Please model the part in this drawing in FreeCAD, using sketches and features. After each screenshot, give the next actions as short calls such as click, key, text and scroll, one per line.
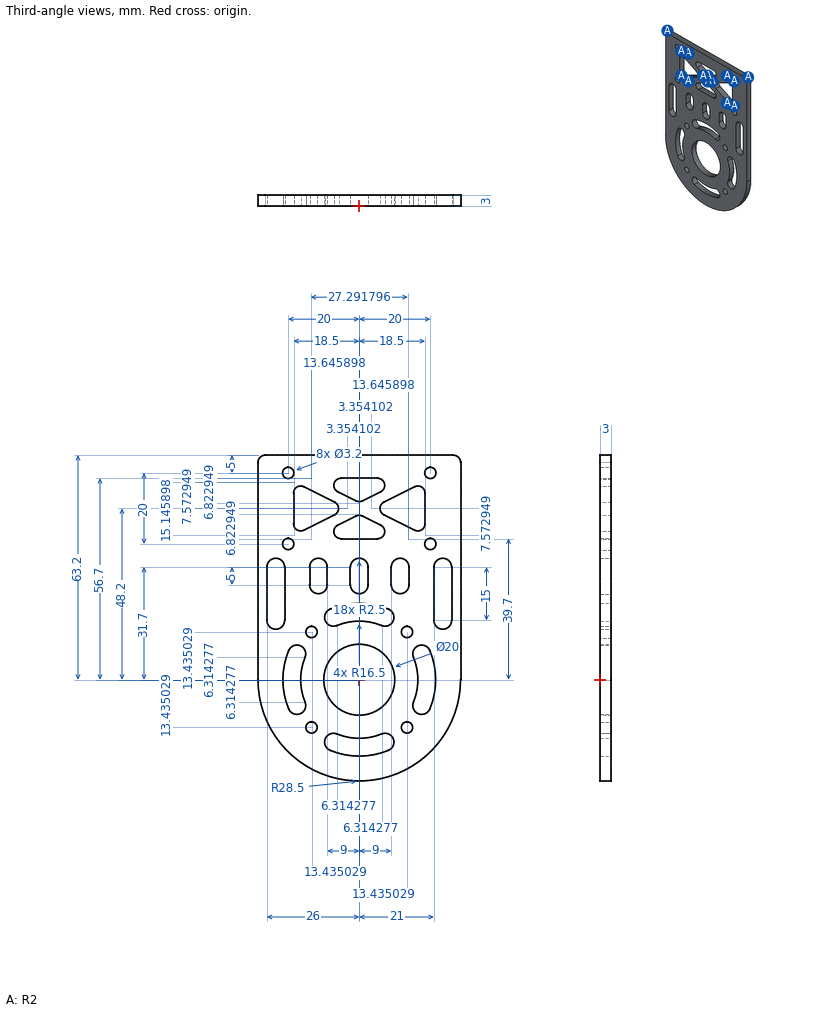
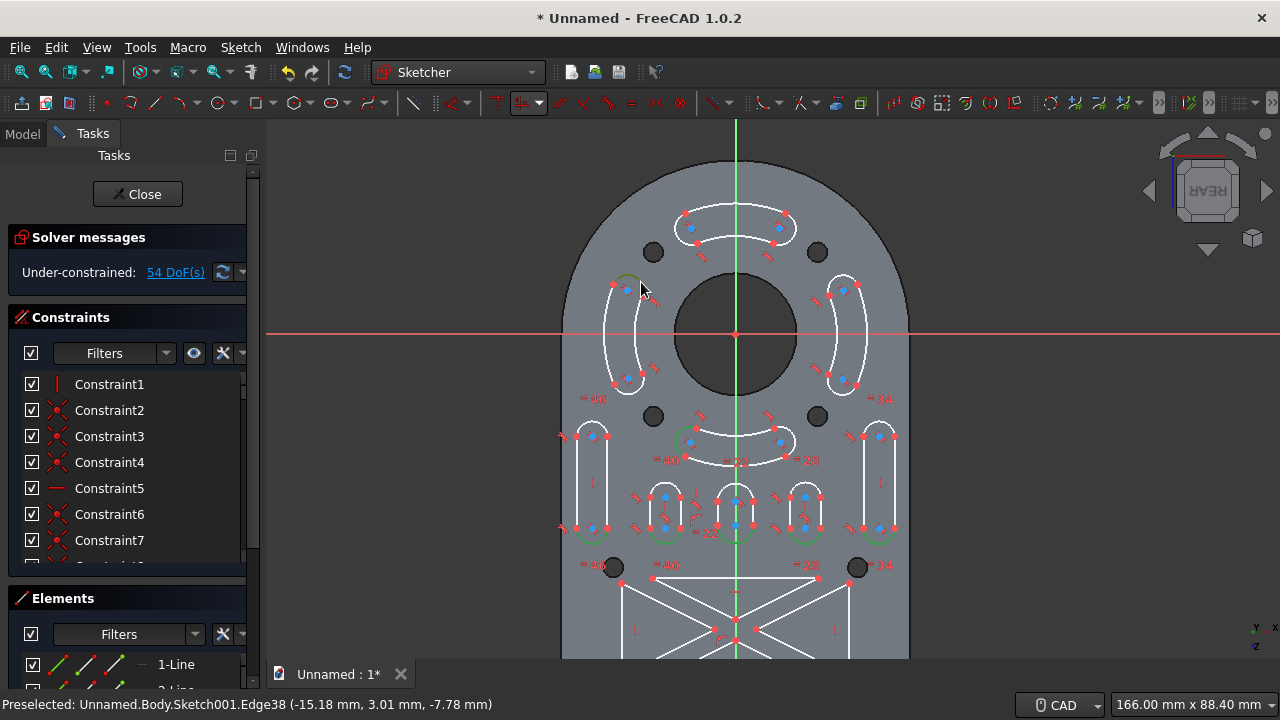
click(830, 388)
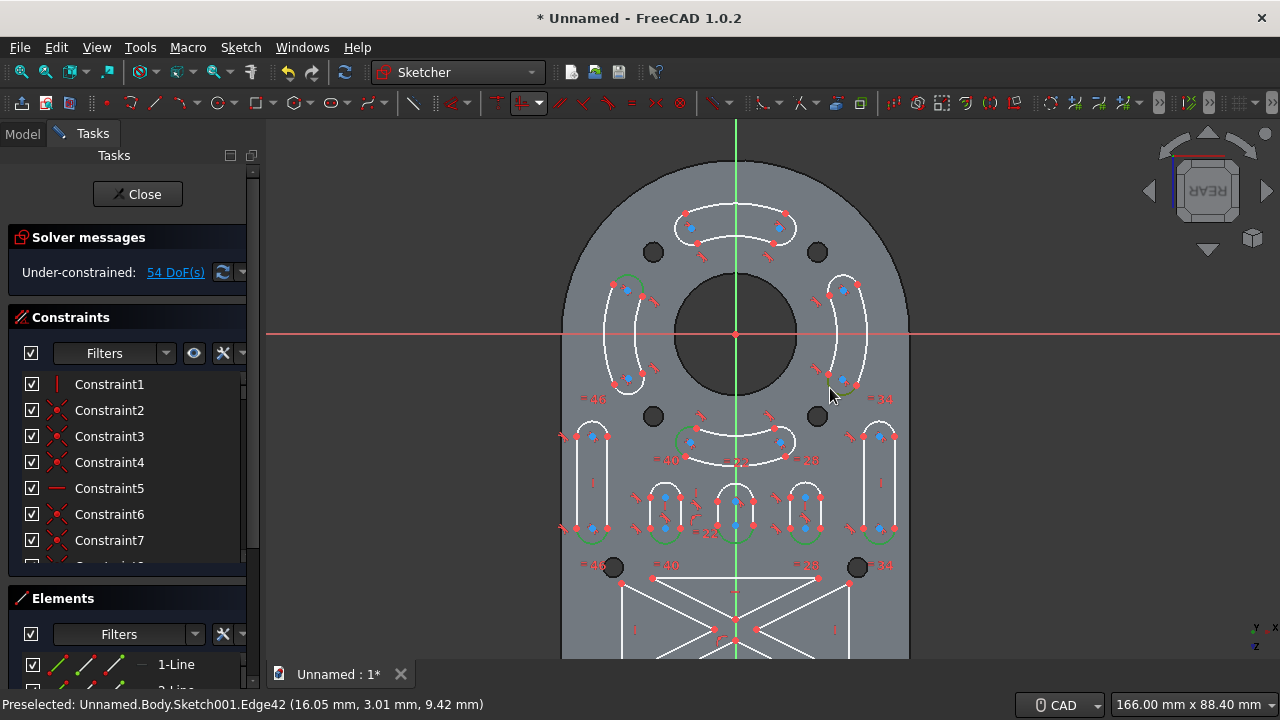
click(788, 242)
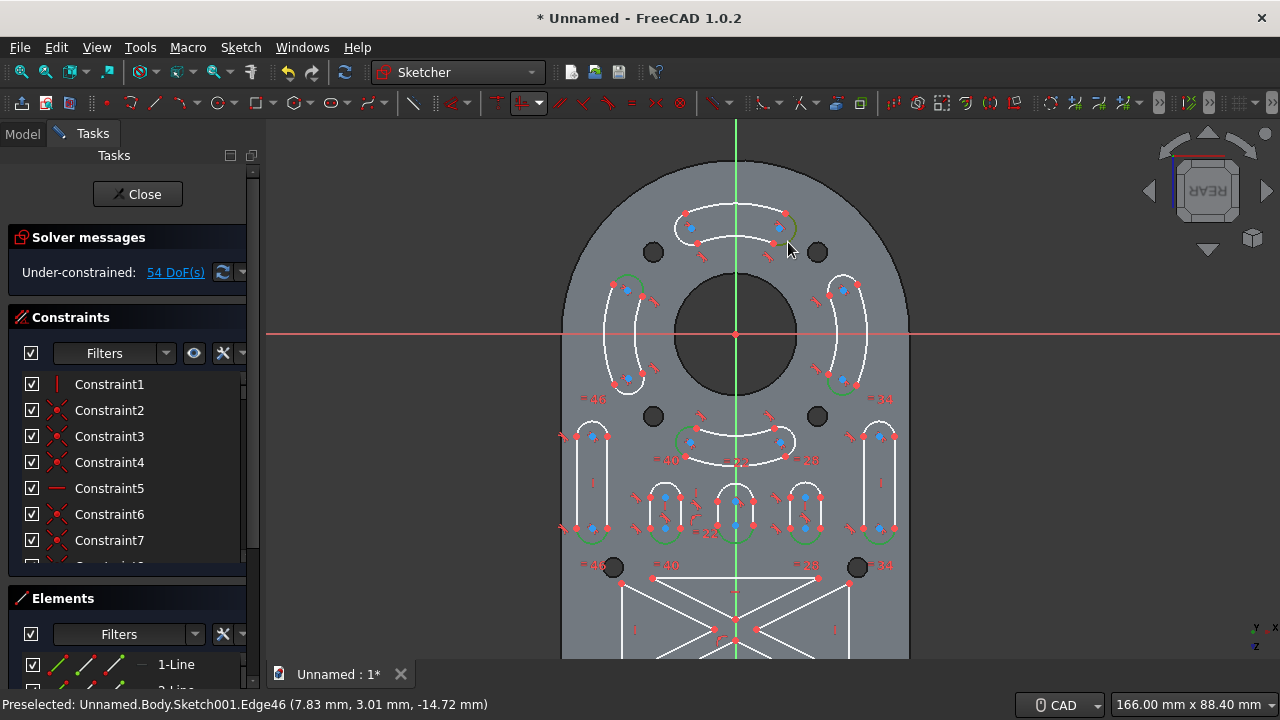
key(e)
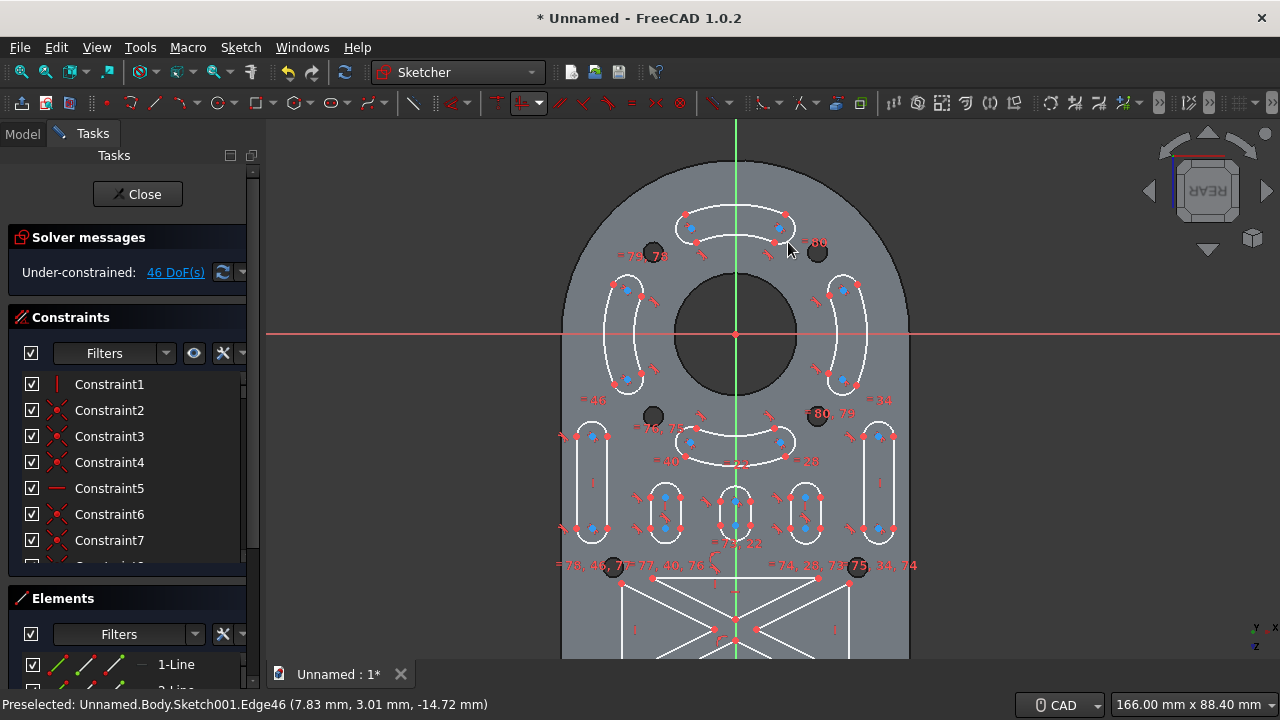
click(720, 435)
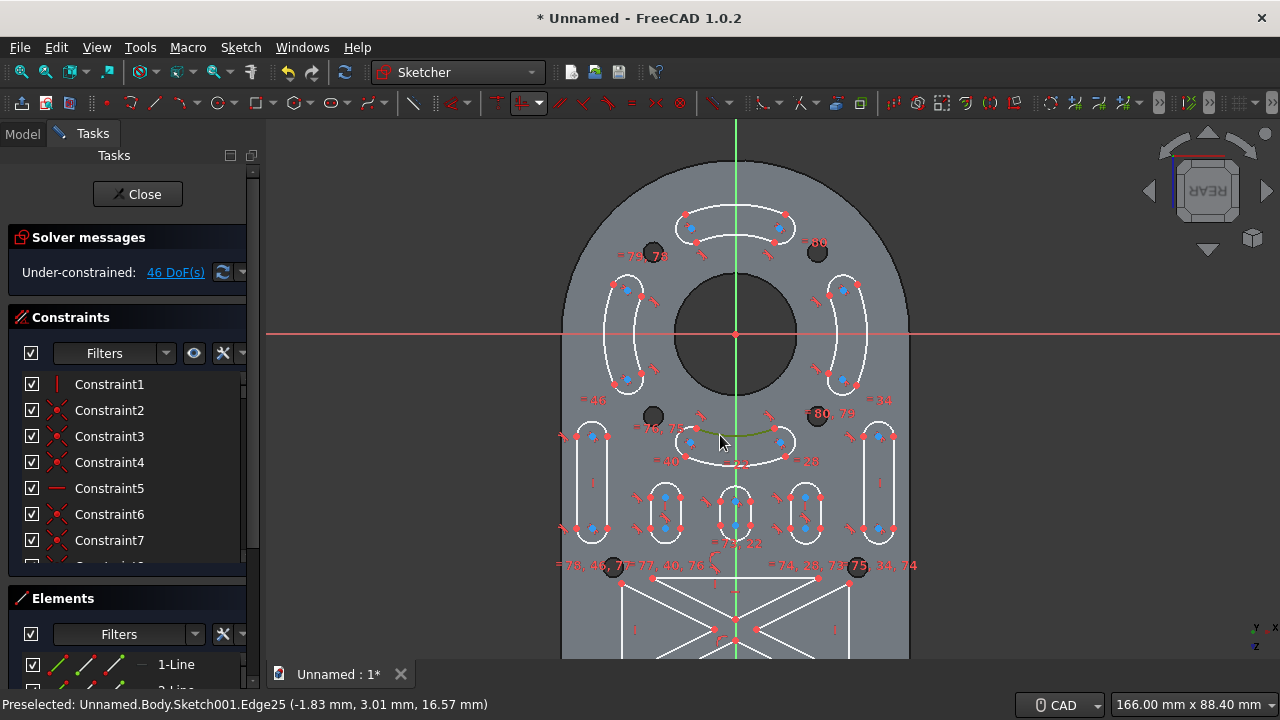
click(635, 319)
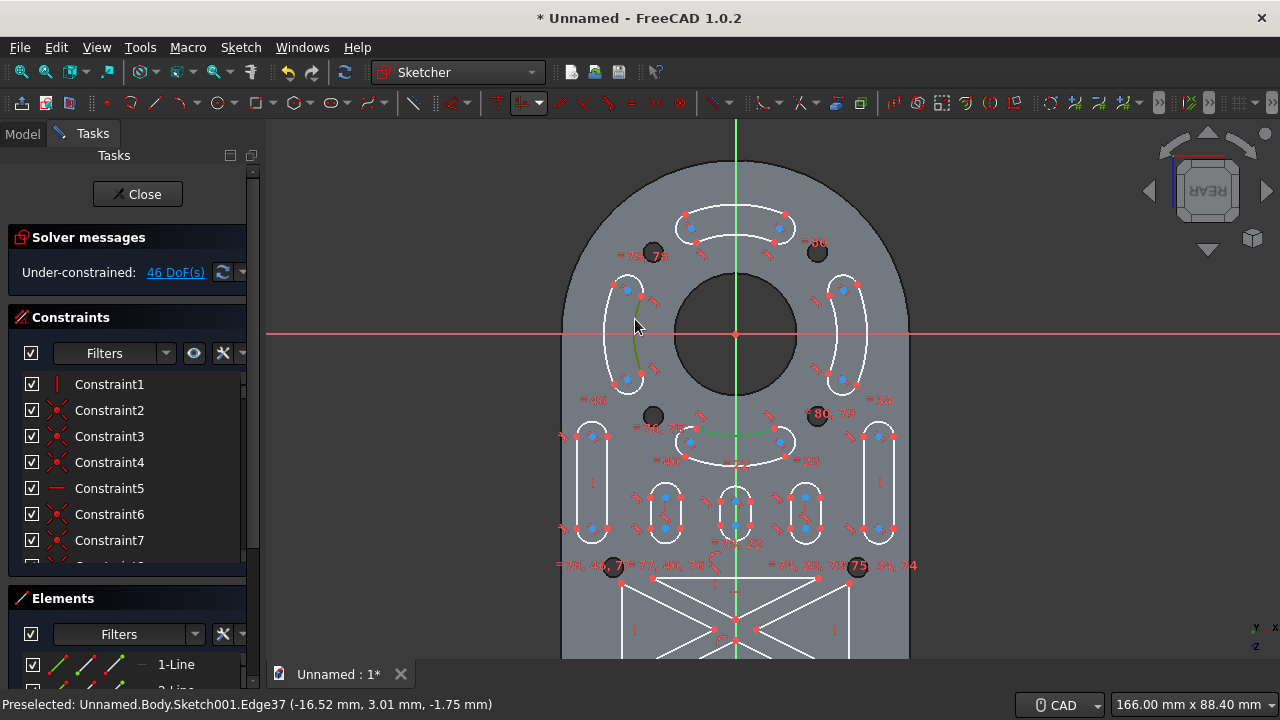
click(836, 351)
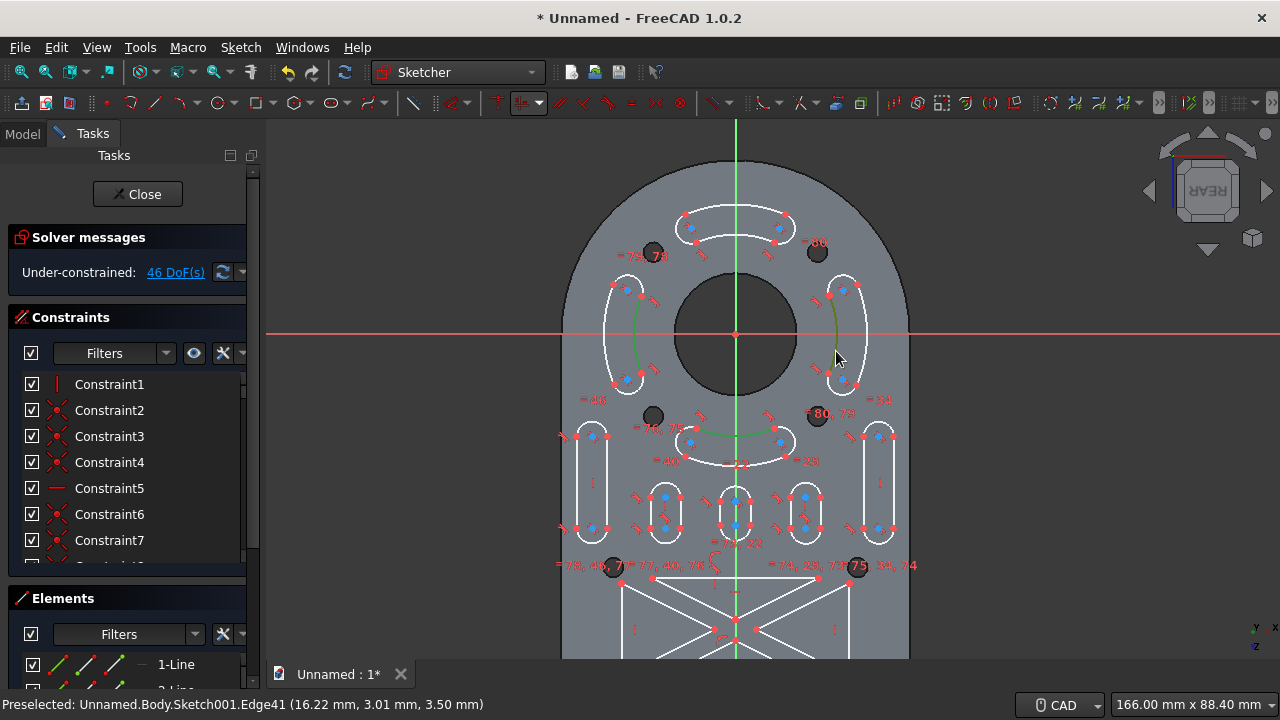
click(751, 236)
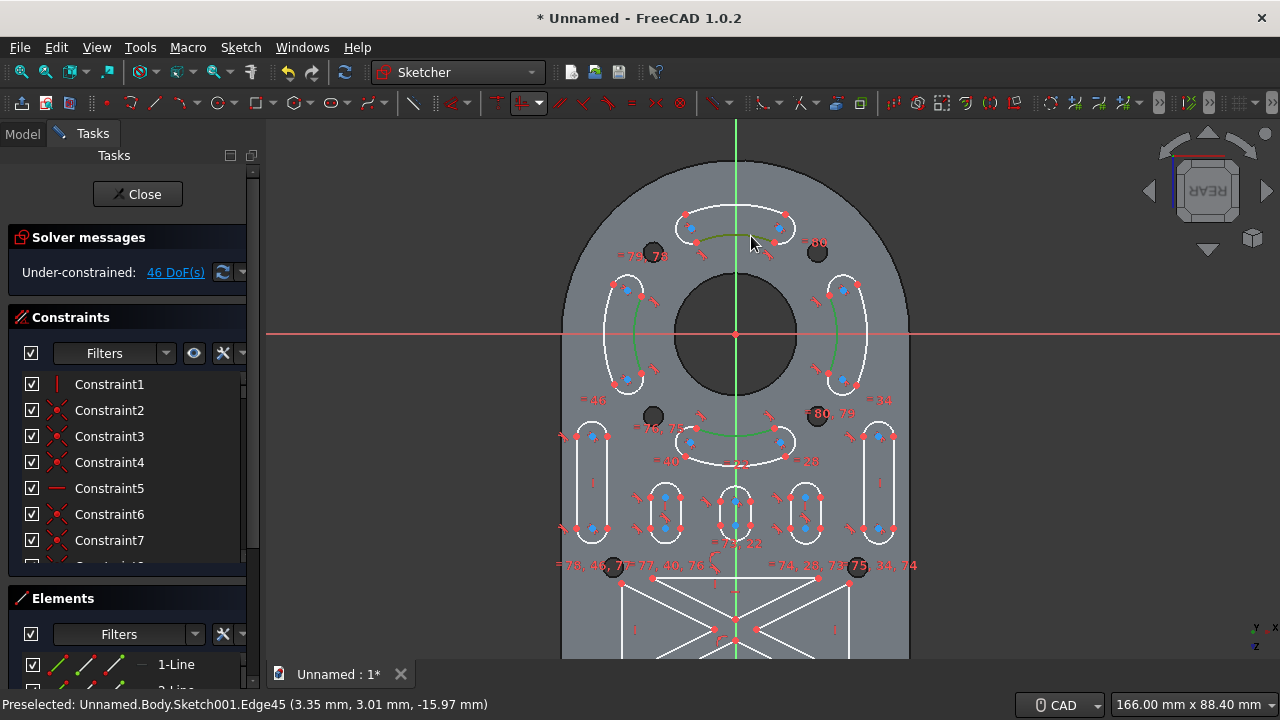
click(632, 104)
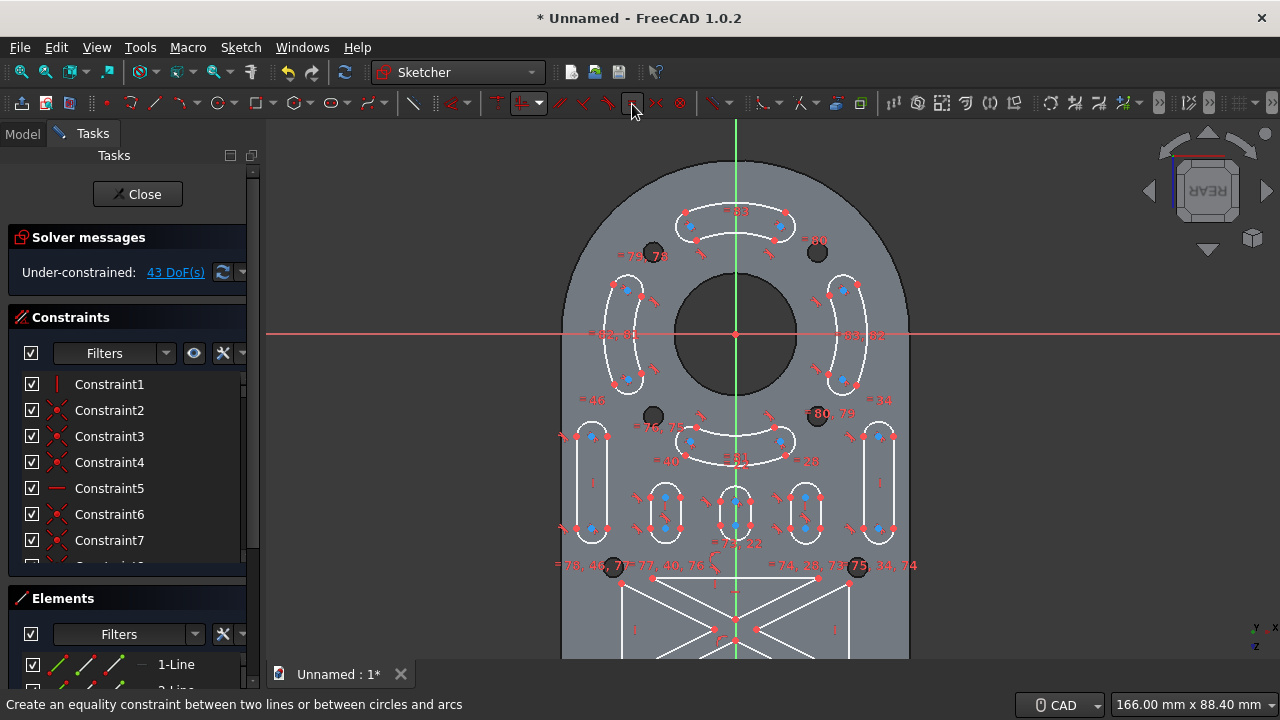
click(452, 104)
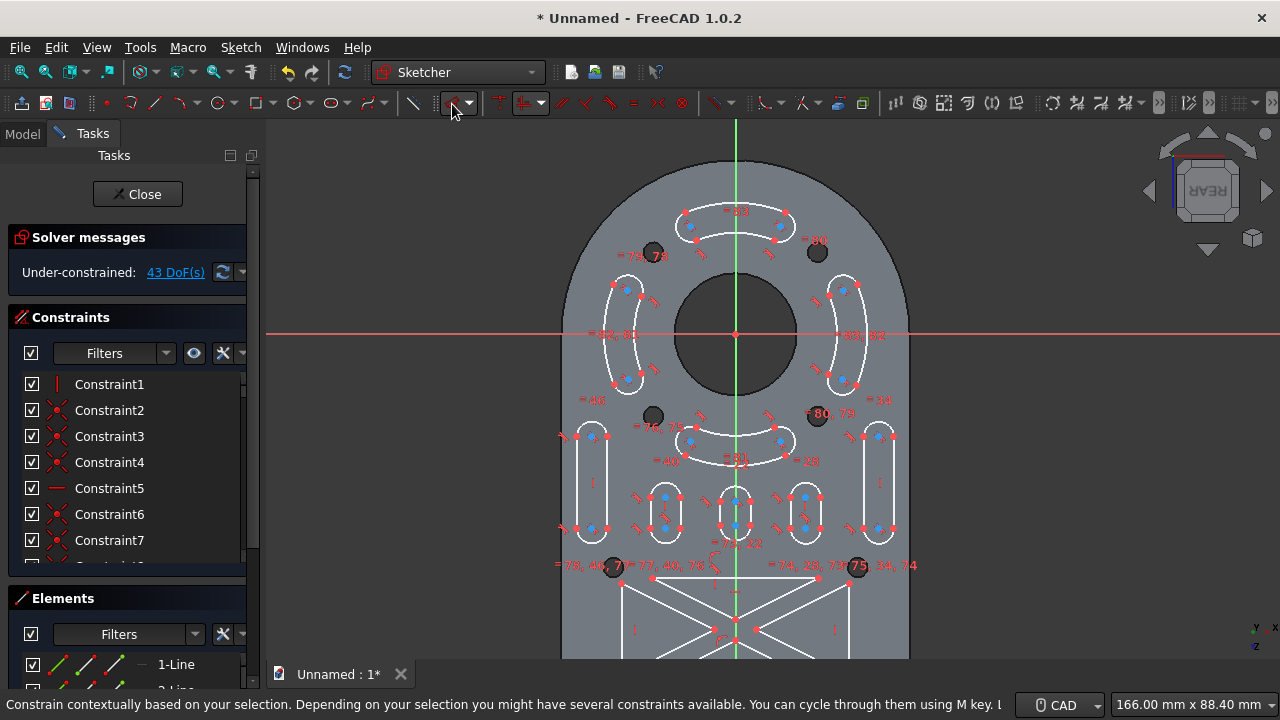
scroll(736, 541, up, 5)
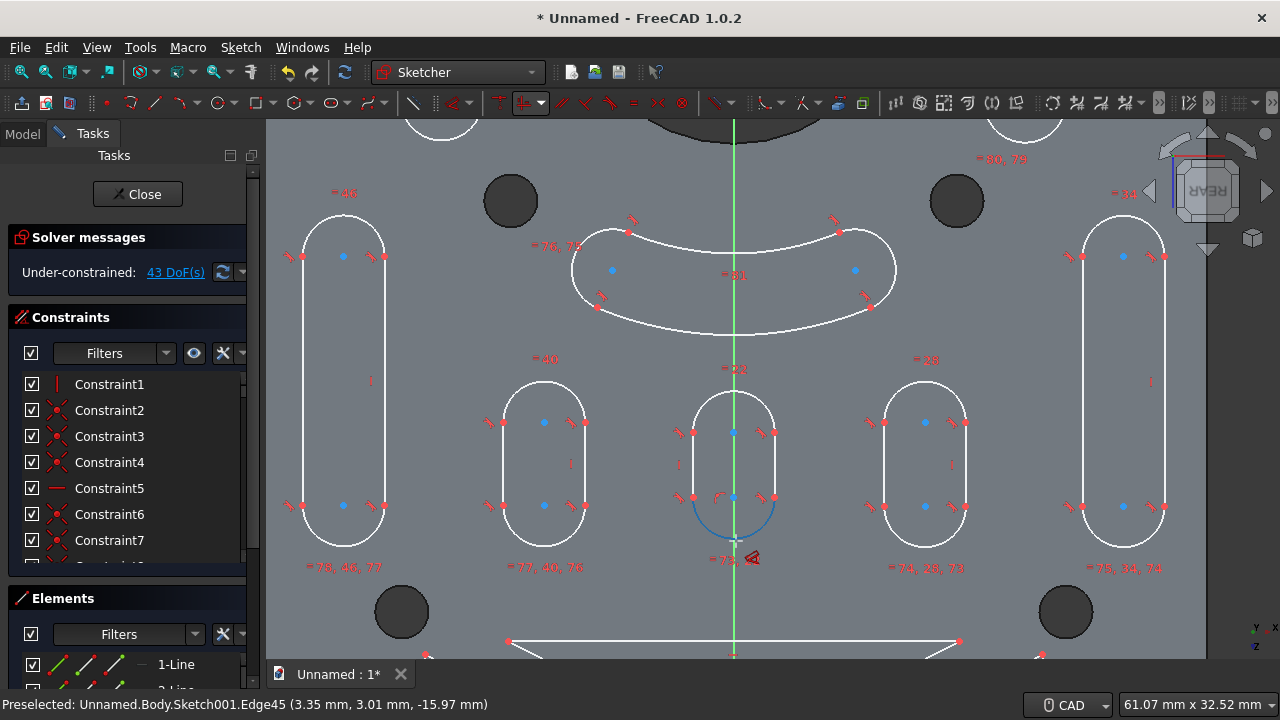
click(734, 539)
click(699, 562)